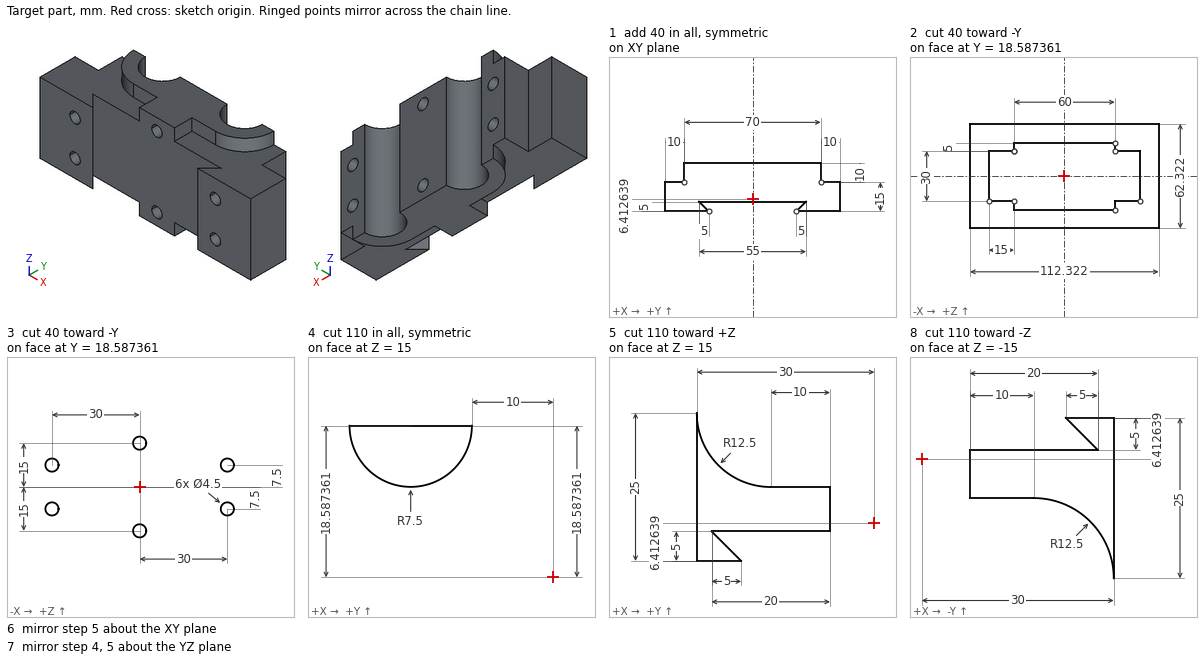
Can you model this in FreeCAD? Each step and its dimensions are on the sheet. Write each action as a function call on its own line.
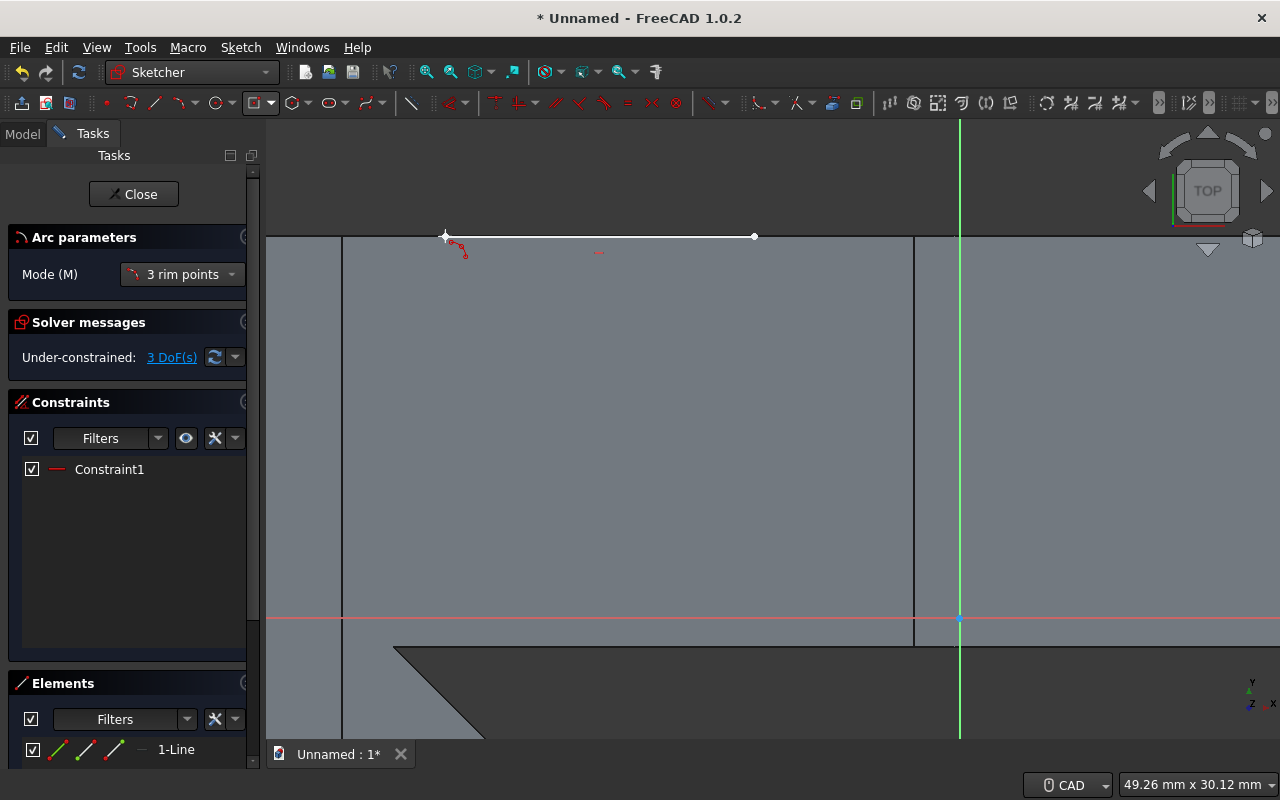
click(445, 237)
click(754, 237)
click(600, 390)
key(Escape)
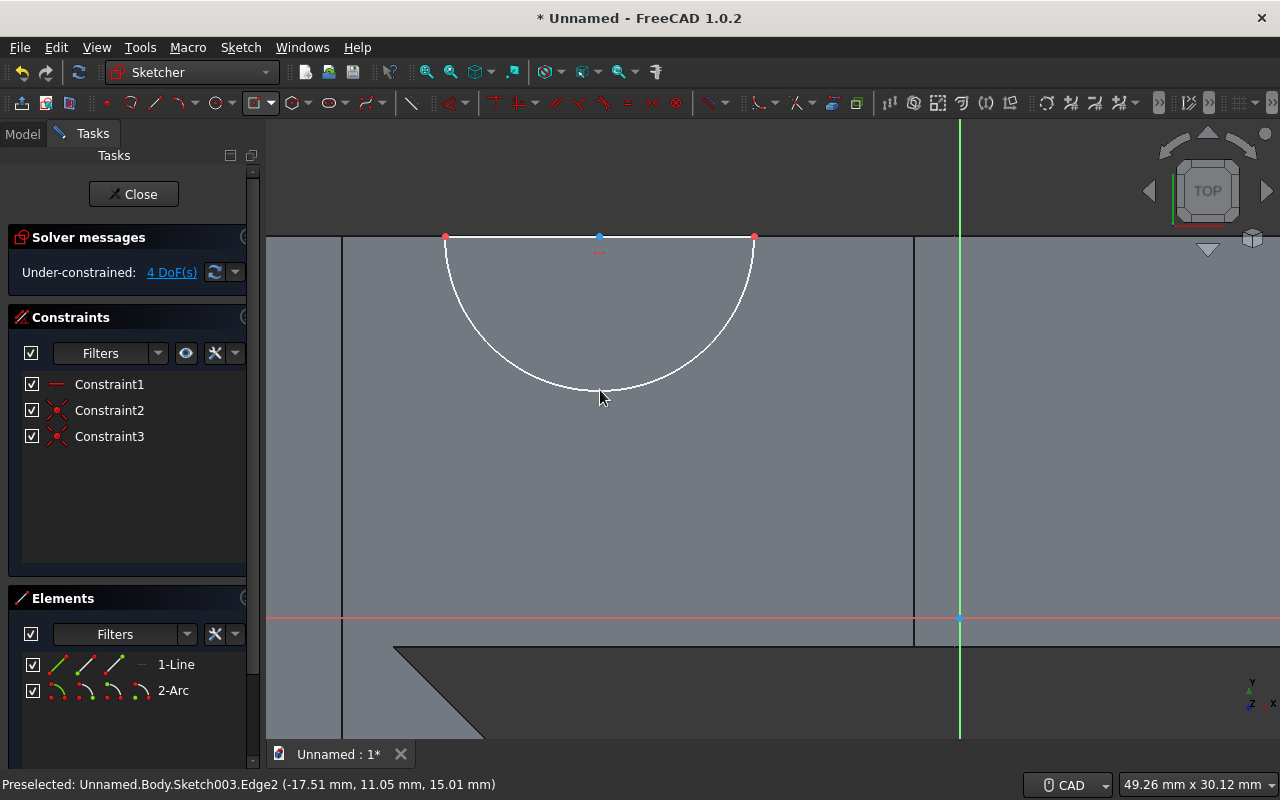
key(d)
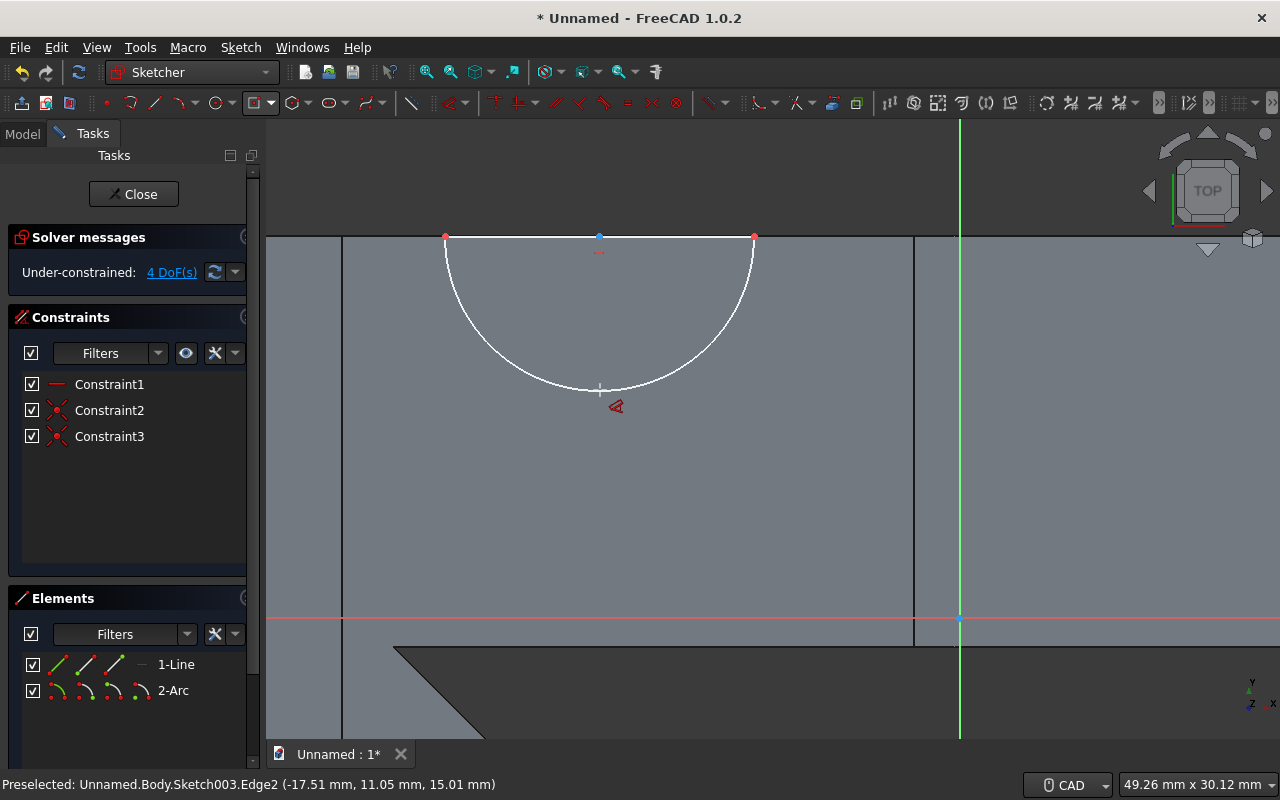
click(509, 362)
click(490, 388)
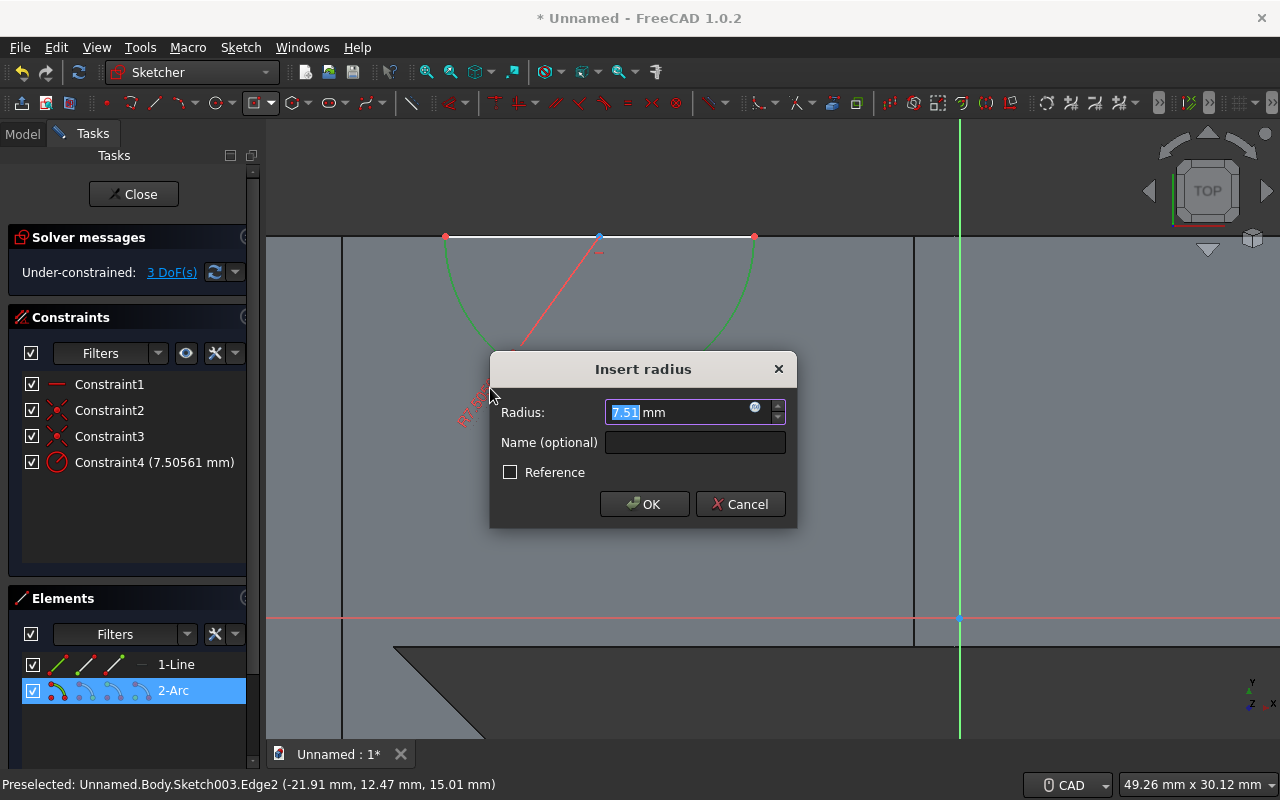
text(7.5)
key(Return)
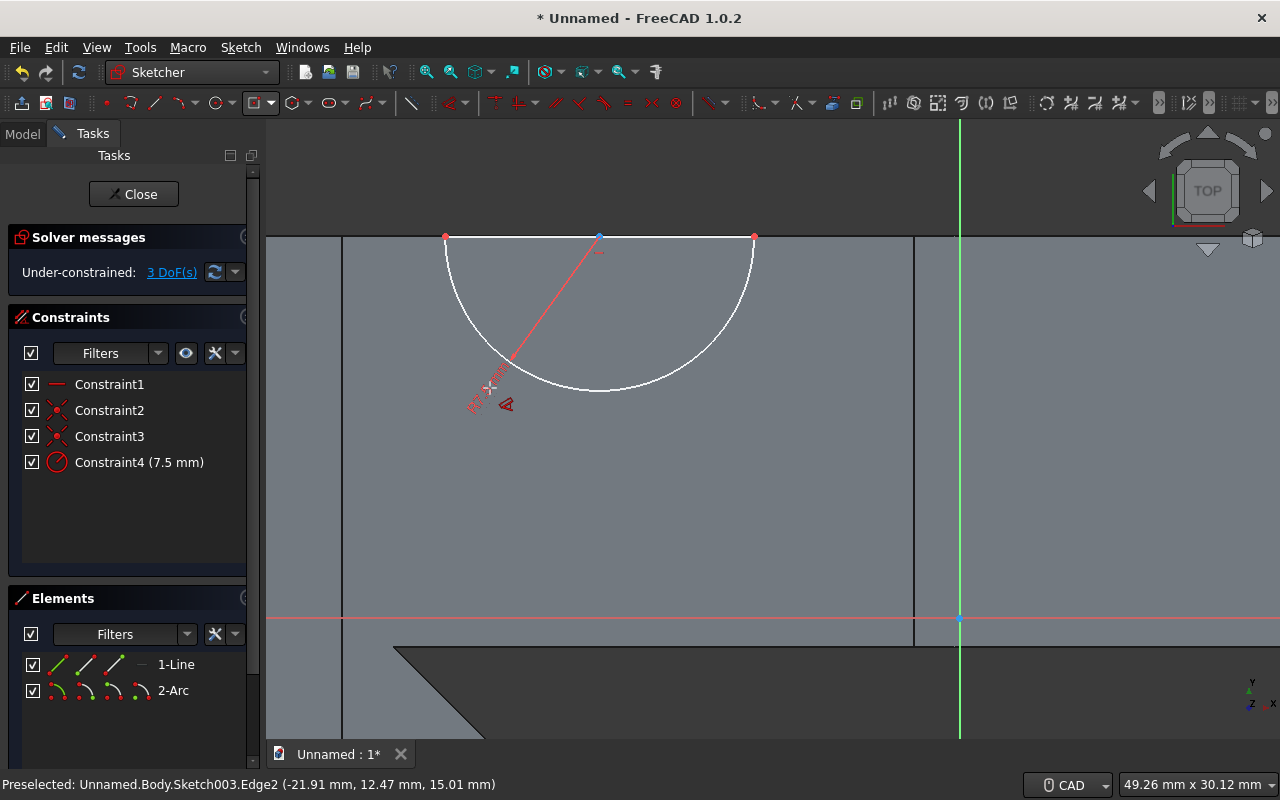
click(754, 237)
click(857, 652)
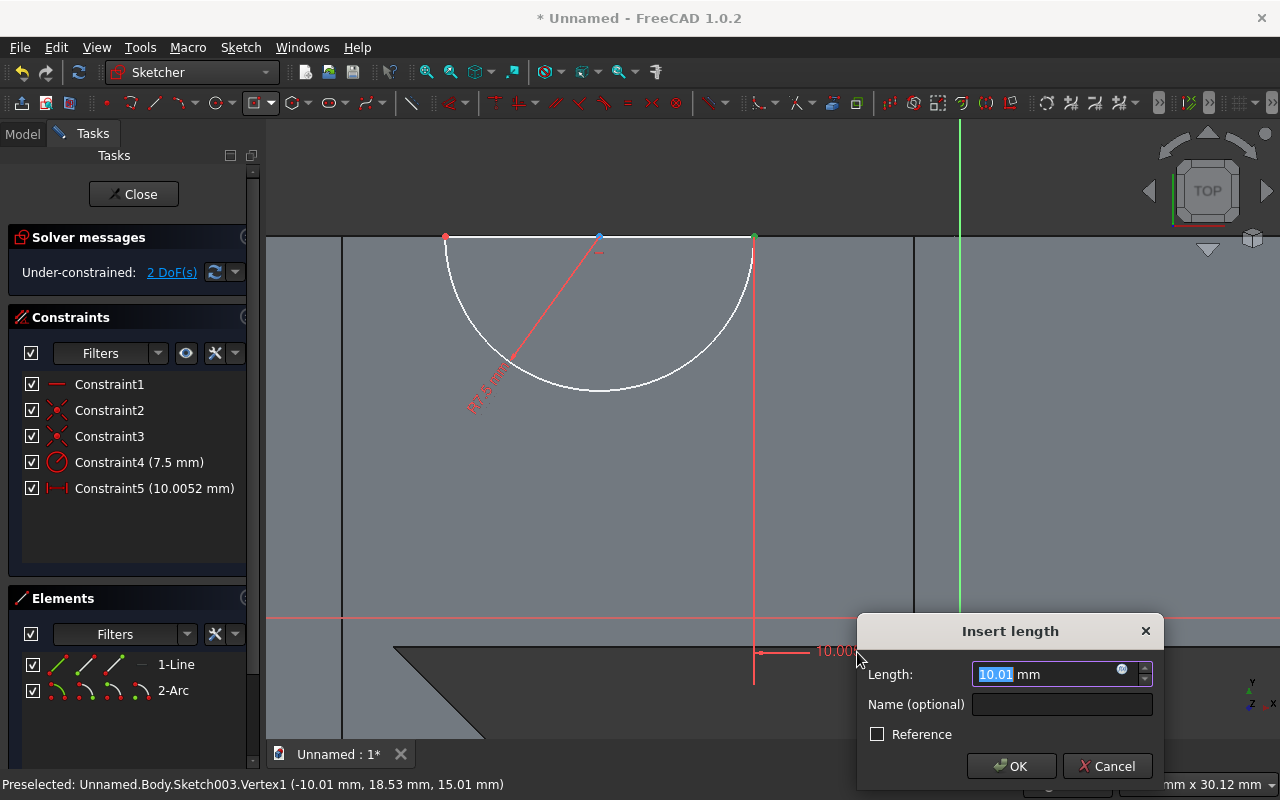
text(10)
key(Return)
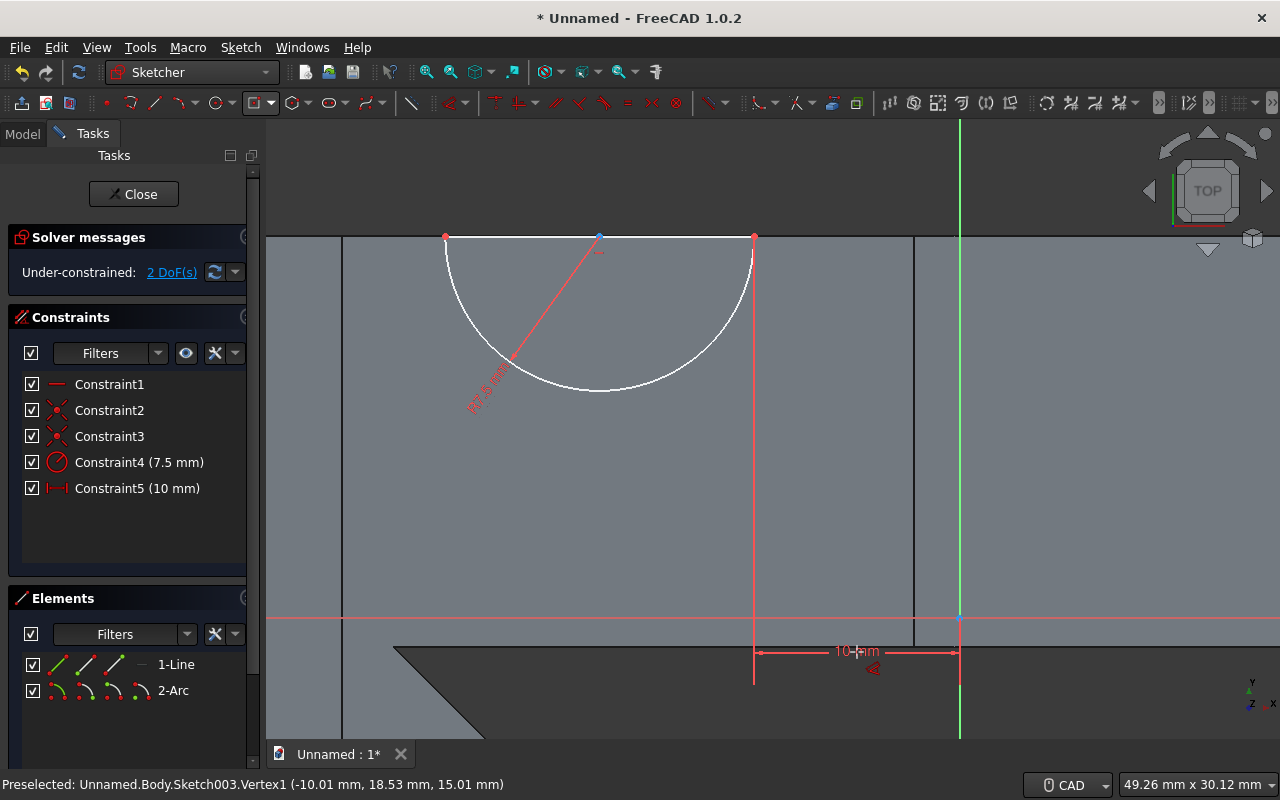
click(754, 237)
click(994, 428)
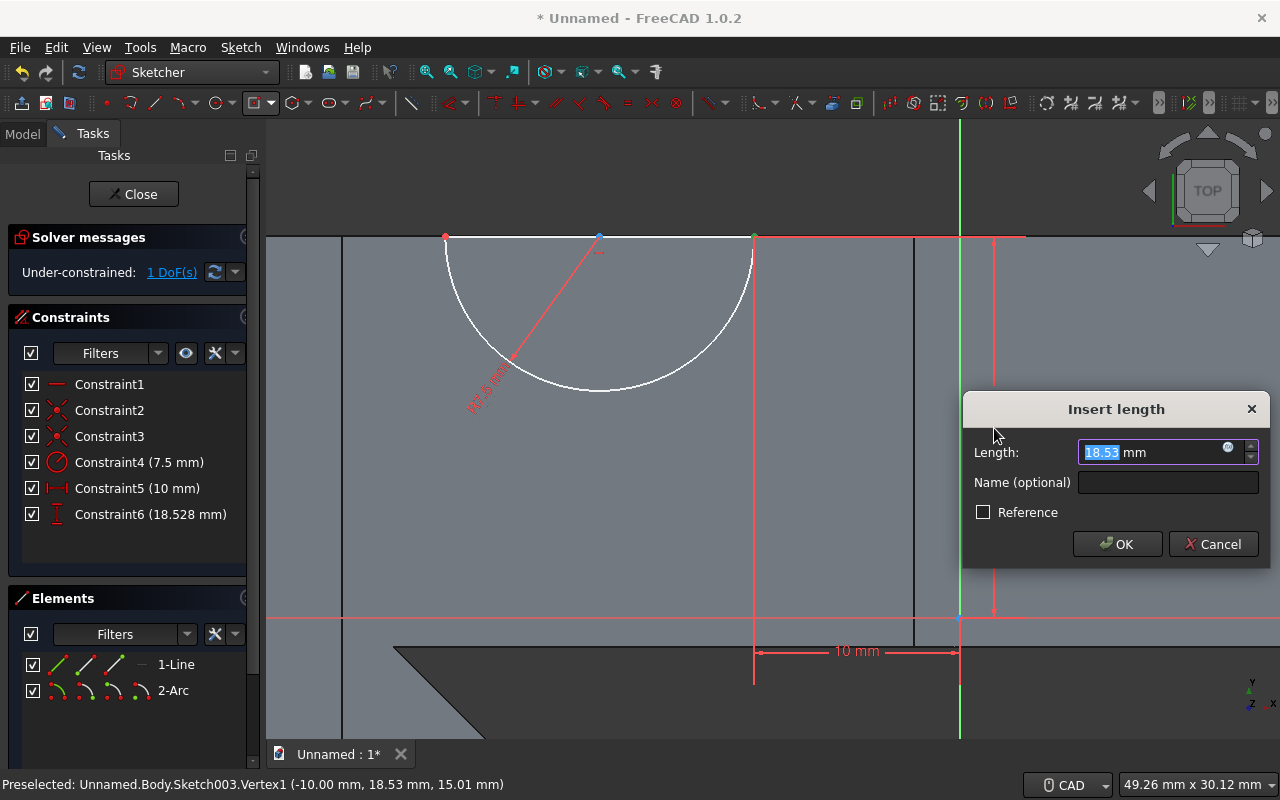
text(18.587361)
key(Return)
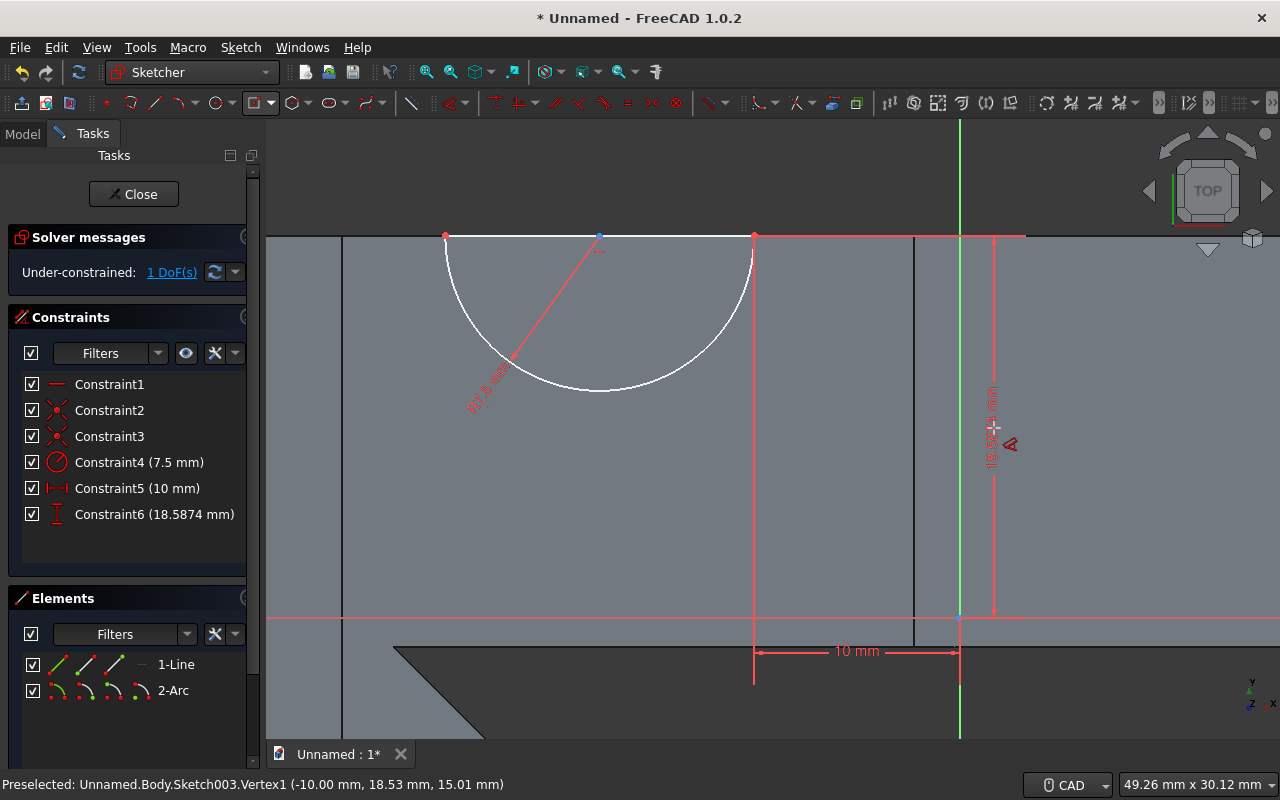
click(600, 237)
click(994, 340)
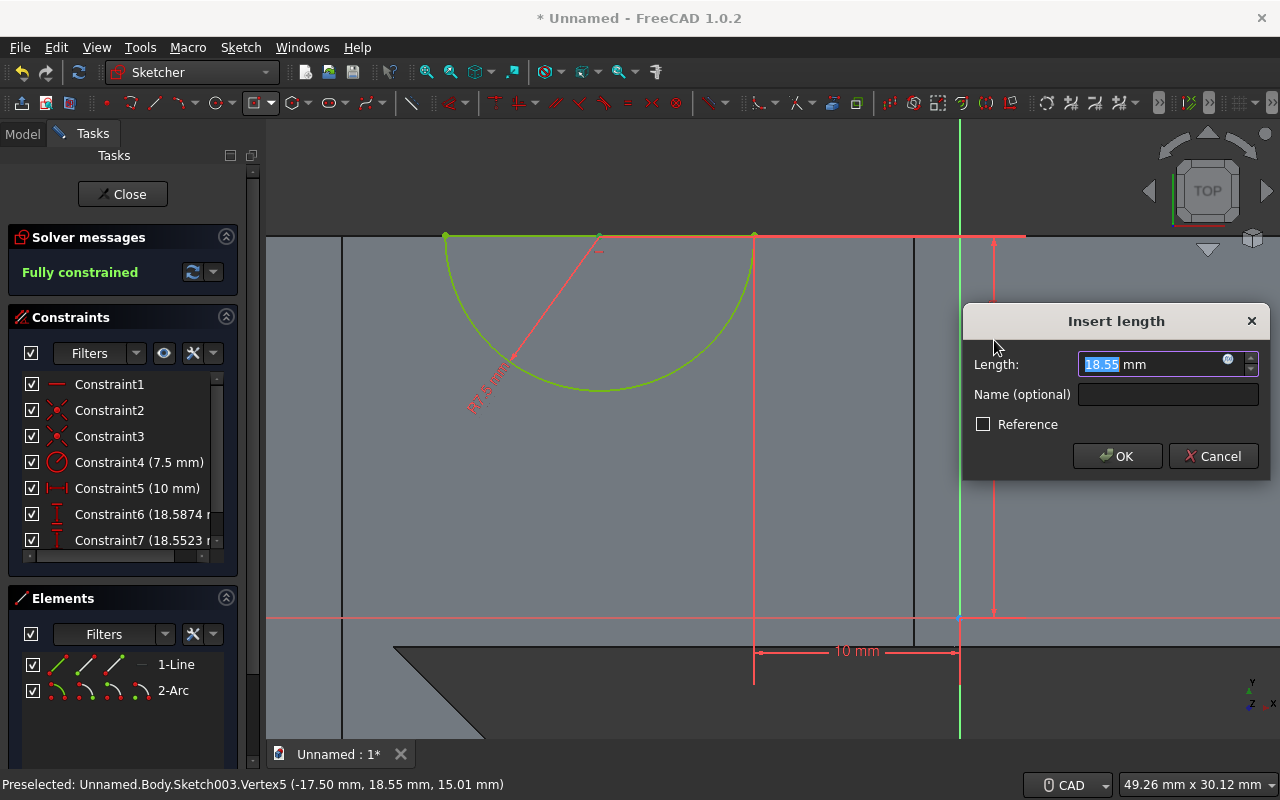
text(18.587361)
key(Return)
key(Escape)